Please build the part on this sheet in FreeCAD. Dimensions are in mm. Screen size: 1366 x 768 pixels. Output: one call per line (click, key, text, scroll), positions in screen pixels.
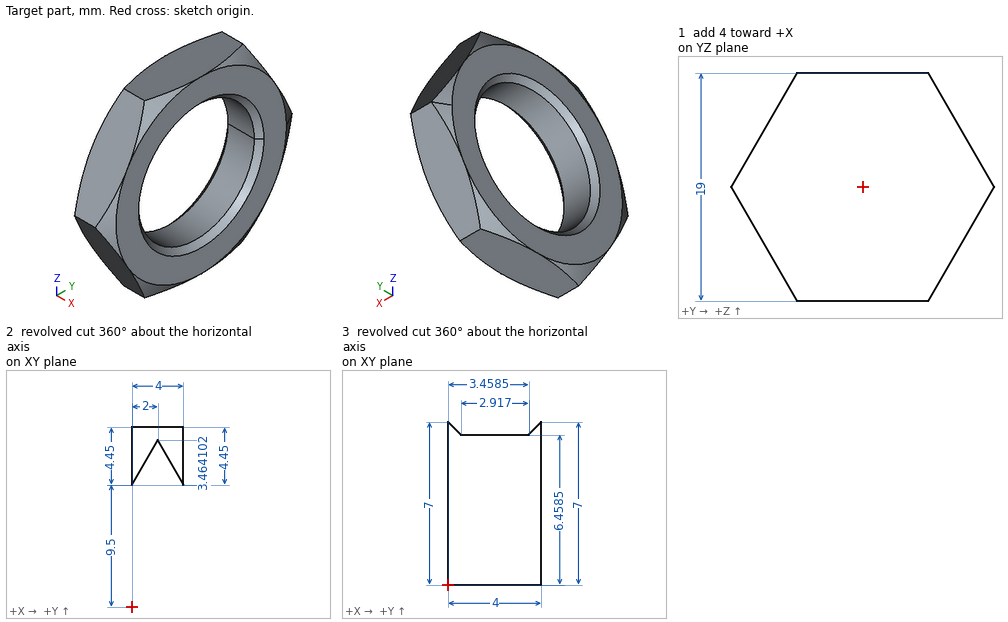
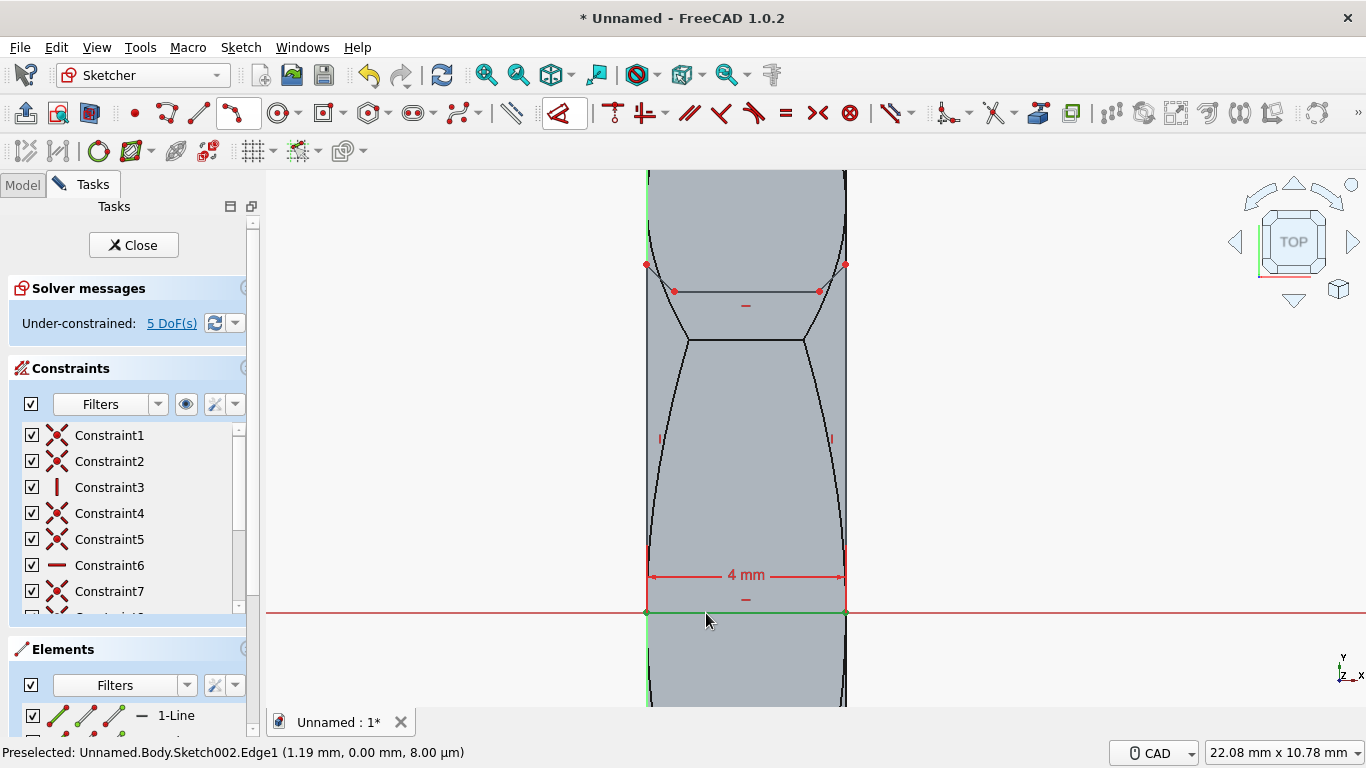
click(846, 509)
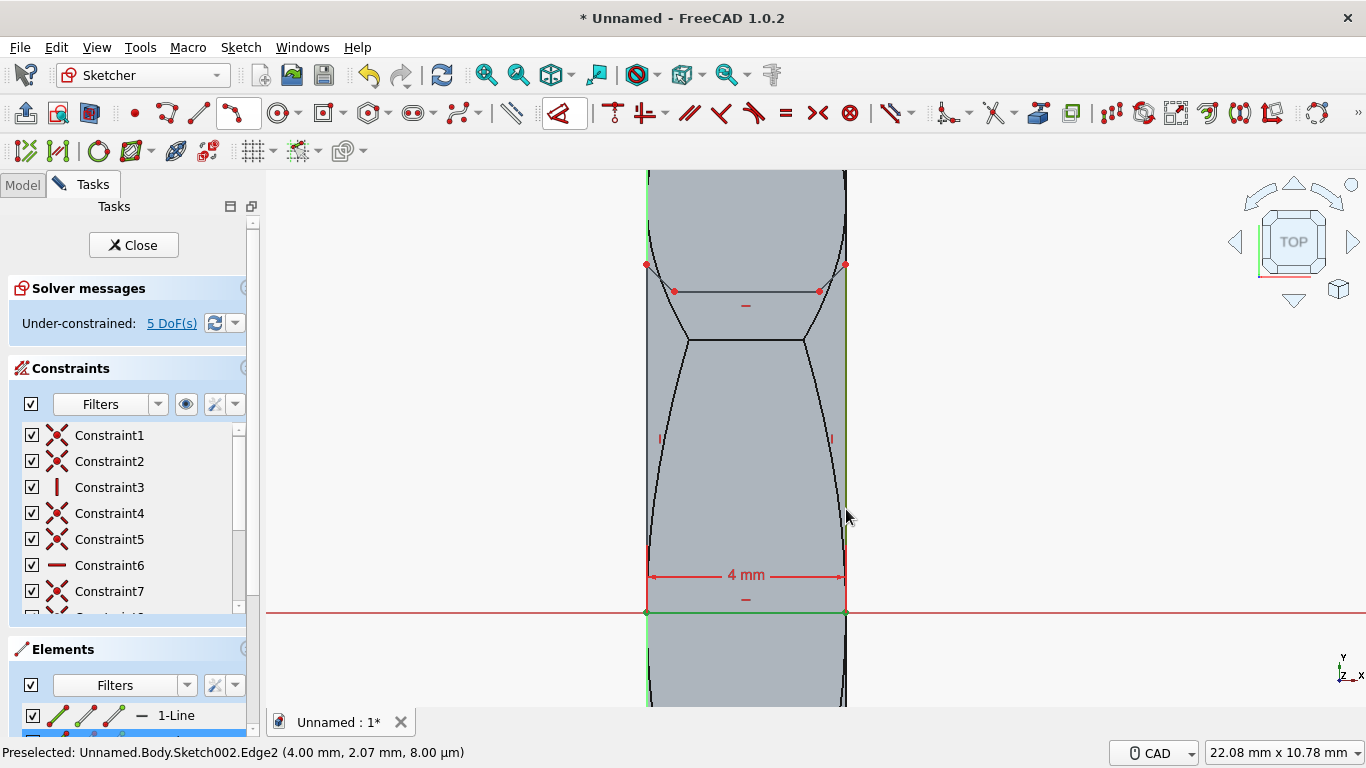
key(i)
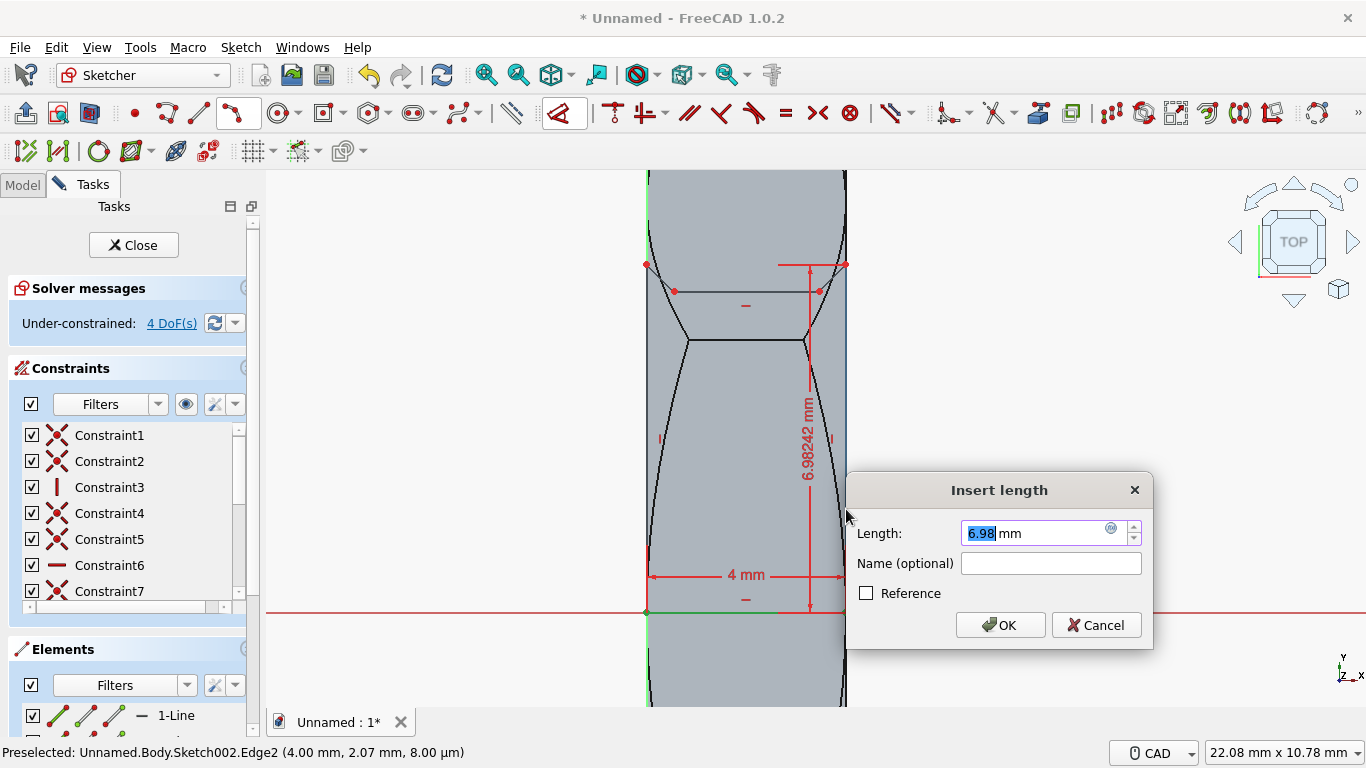
text(7)
key(Return)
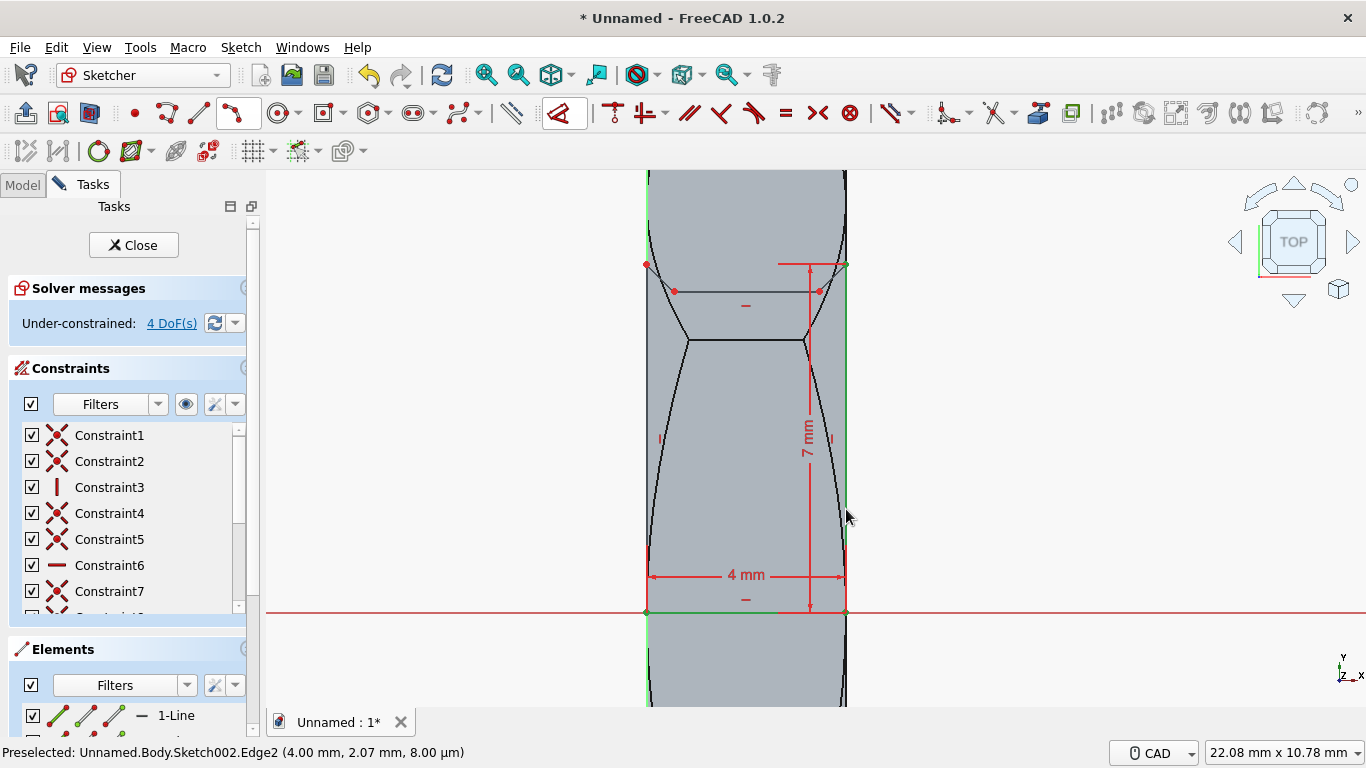
click(647, 369)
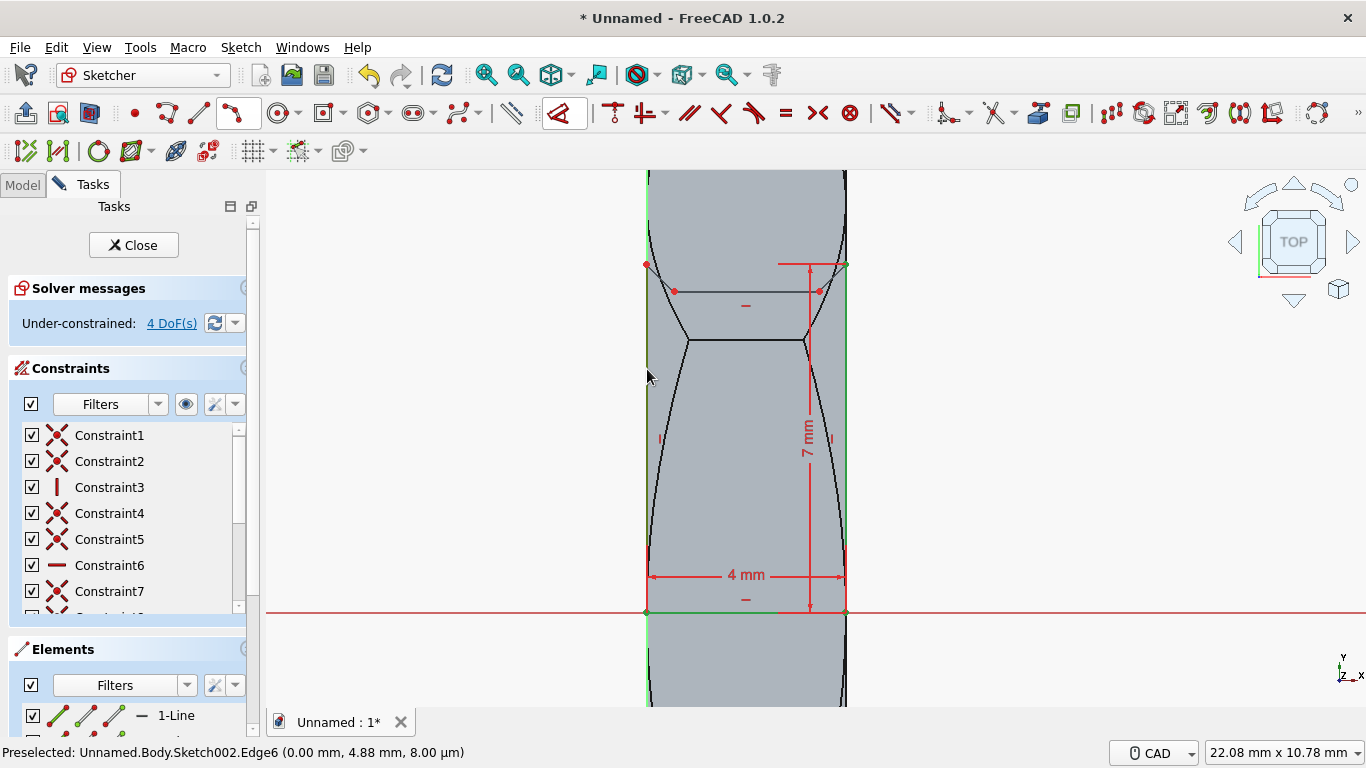
key(i)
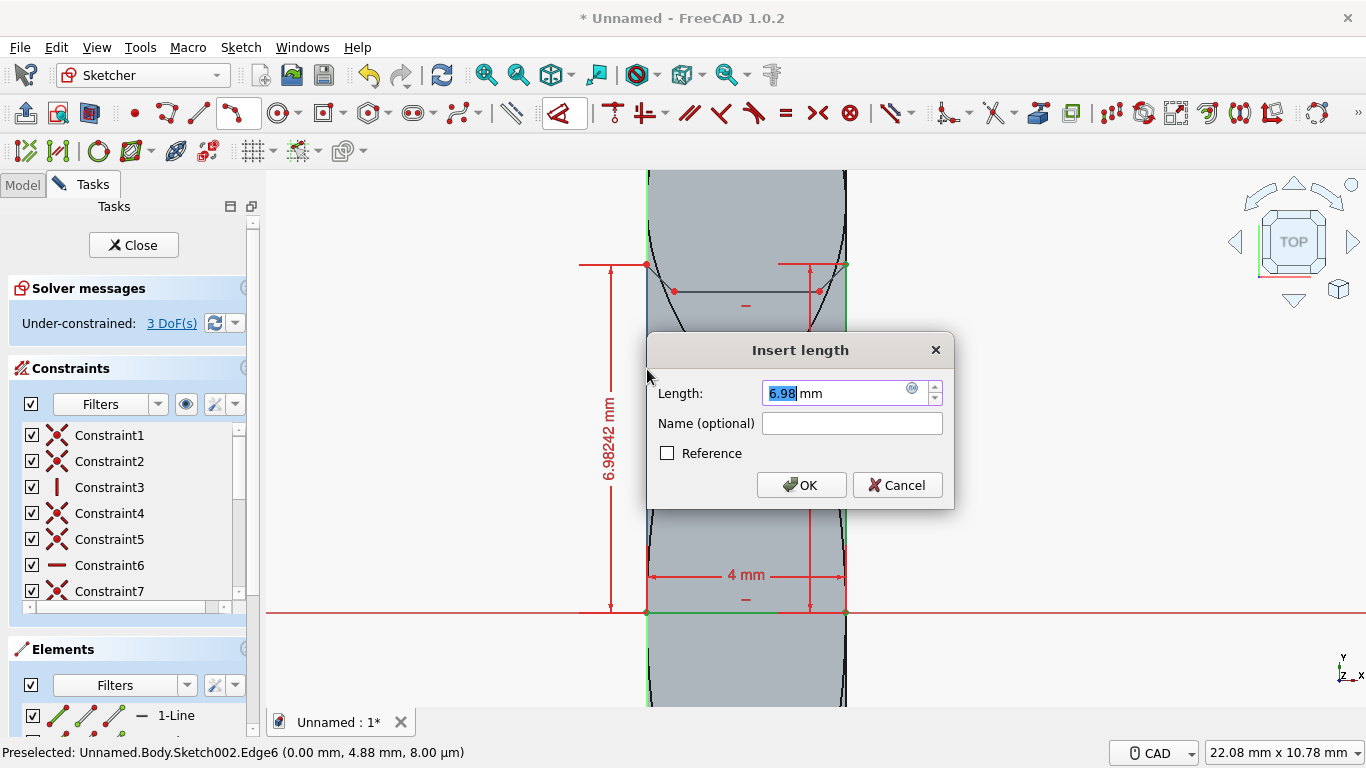
text(7)
key(Return)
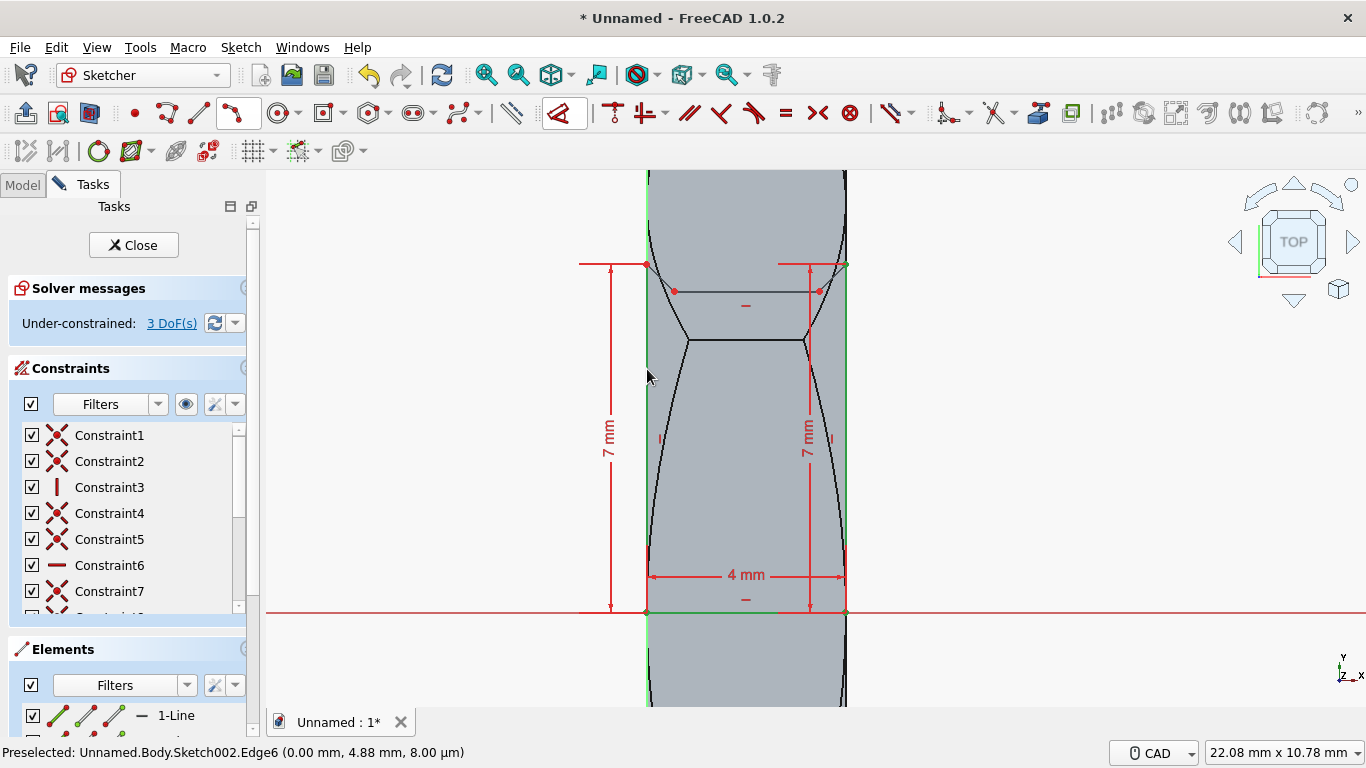
click(776, 292)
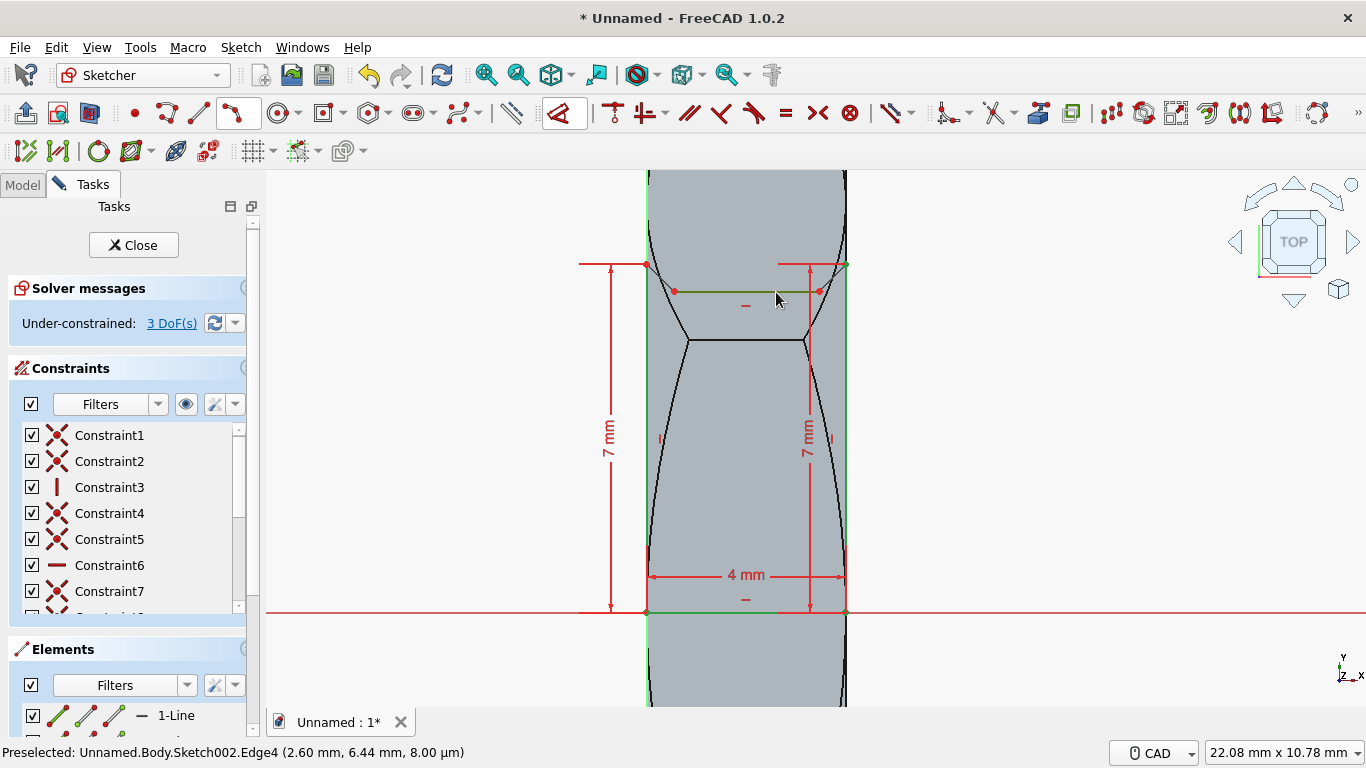
key(l)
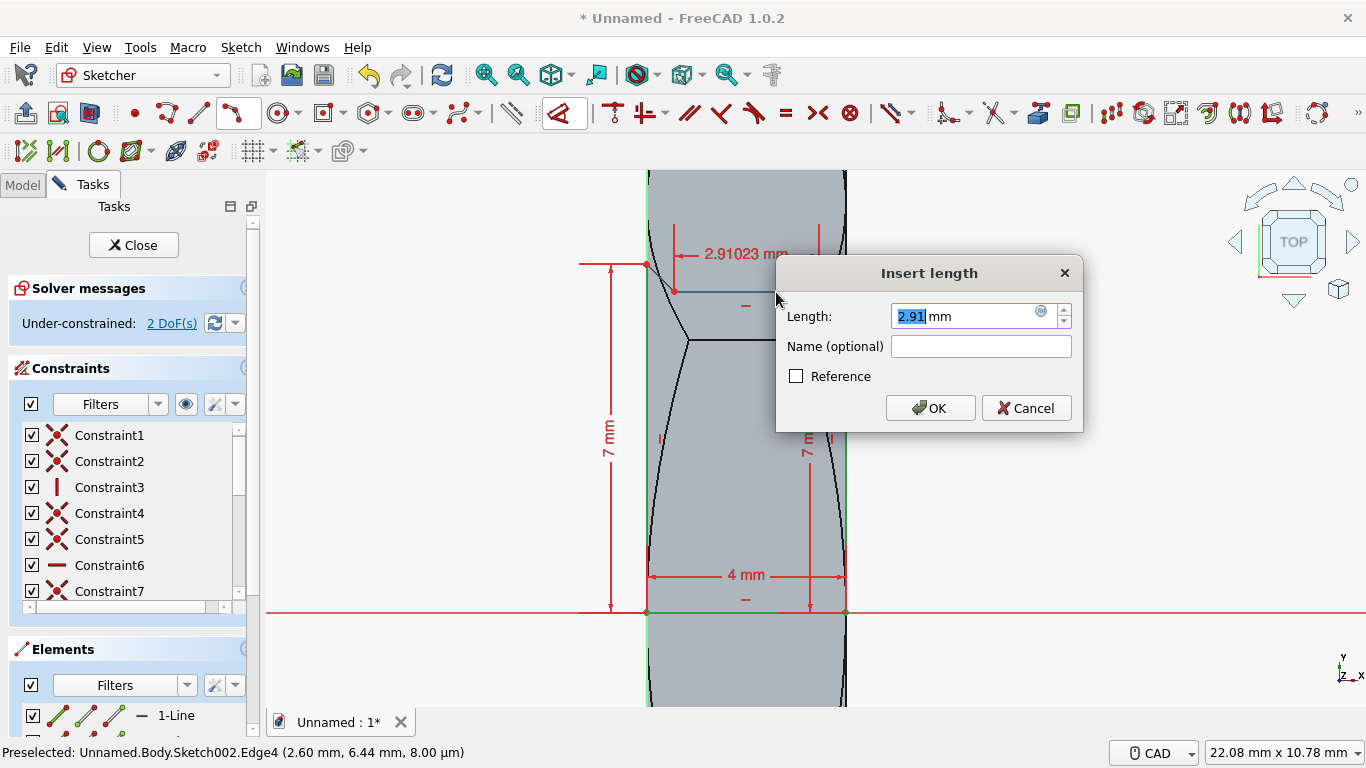
text(2.917)
key(Return)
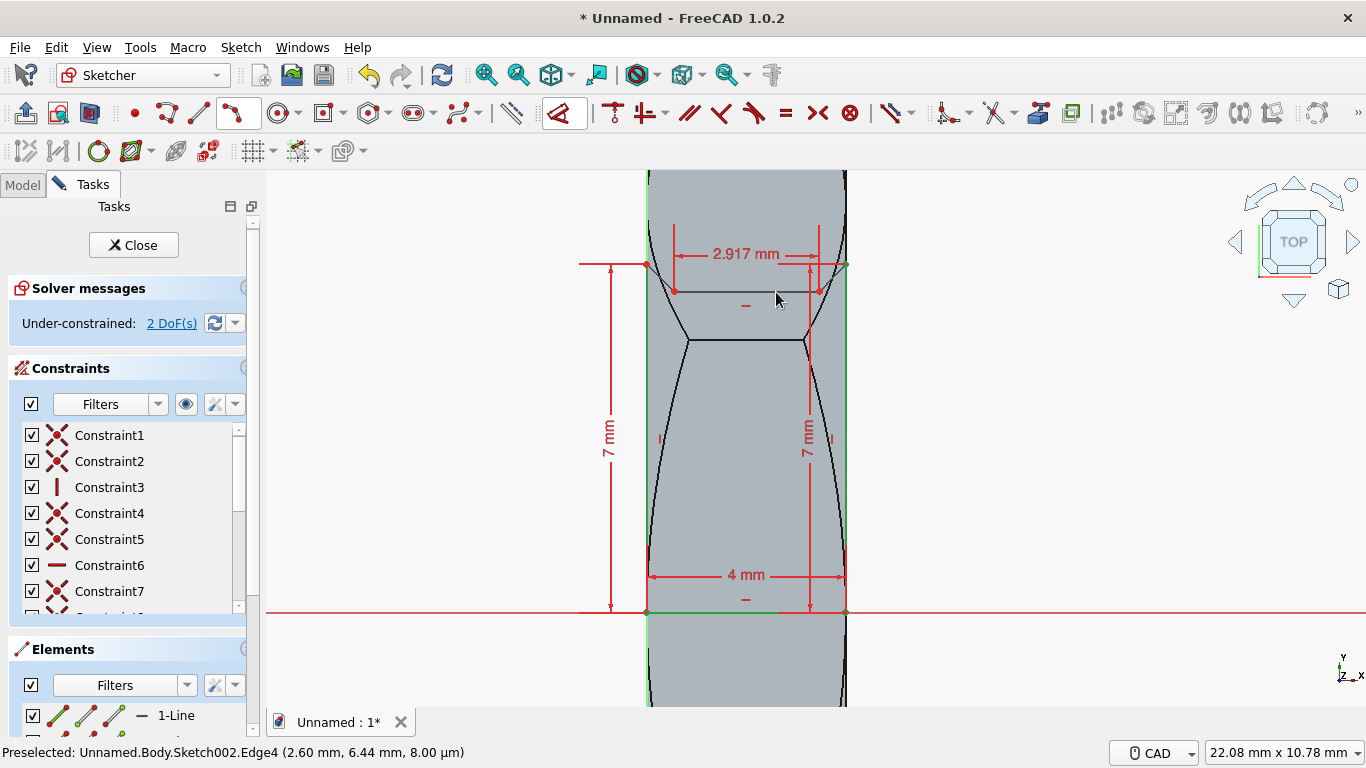
click(819, 292)